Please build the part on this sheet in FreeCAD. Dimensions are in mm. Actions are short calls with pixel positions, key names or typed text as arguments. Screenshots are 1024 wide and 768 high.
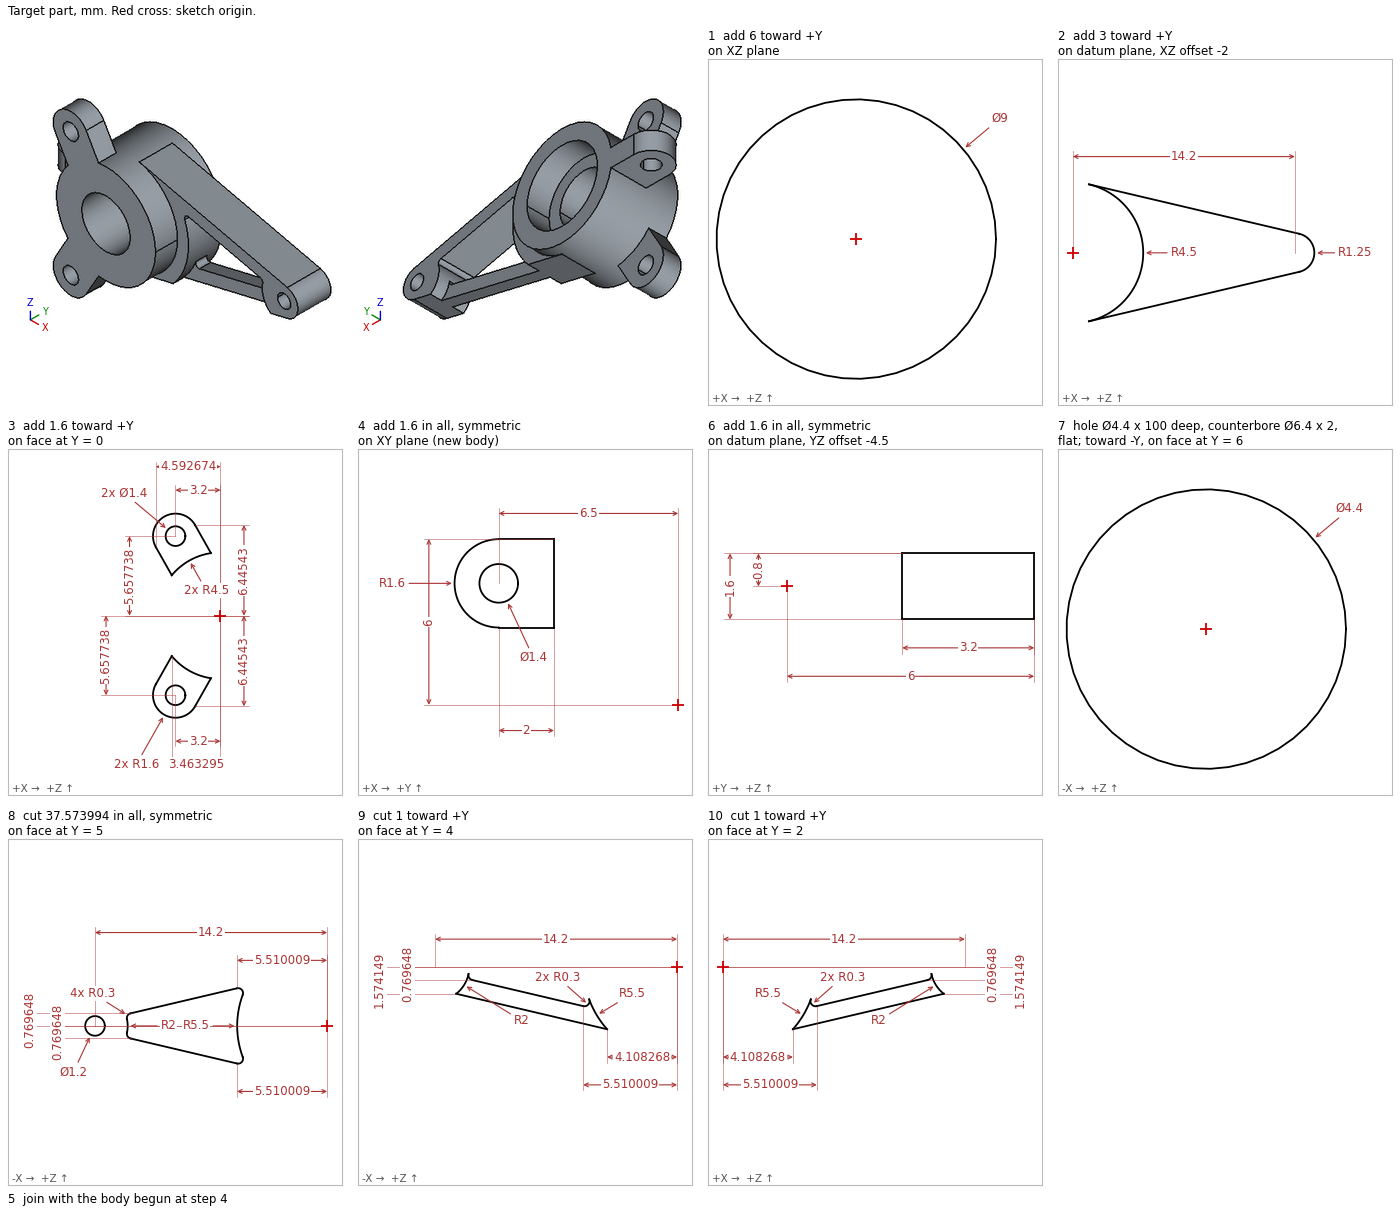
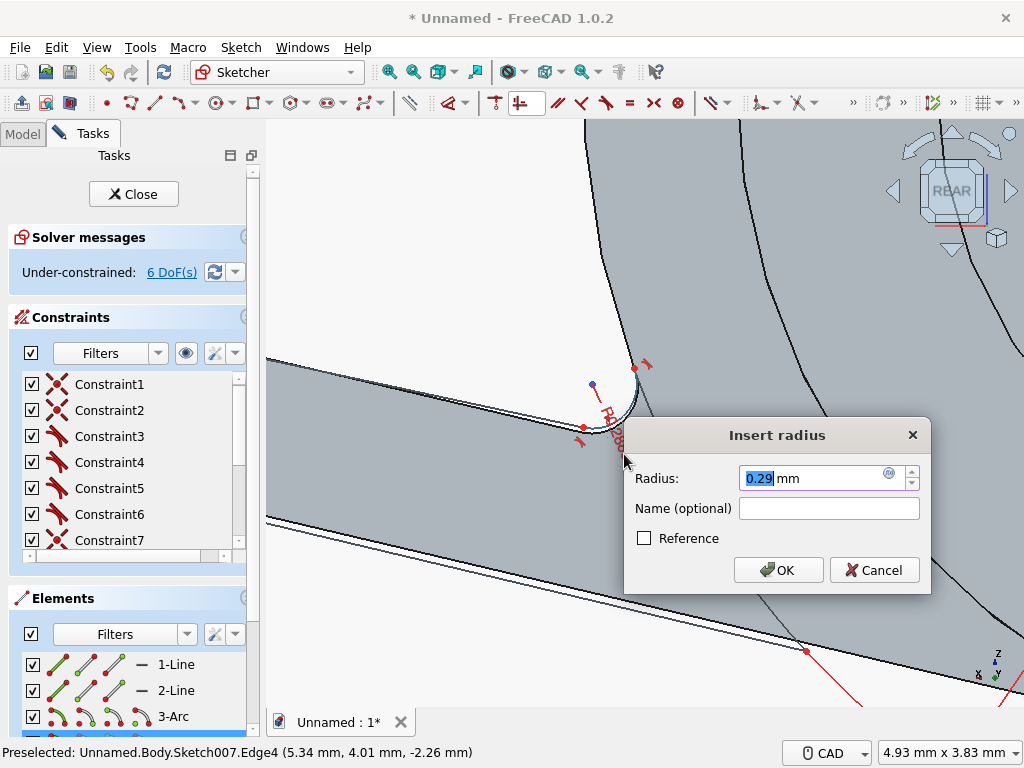
text(0.3)
key(Return)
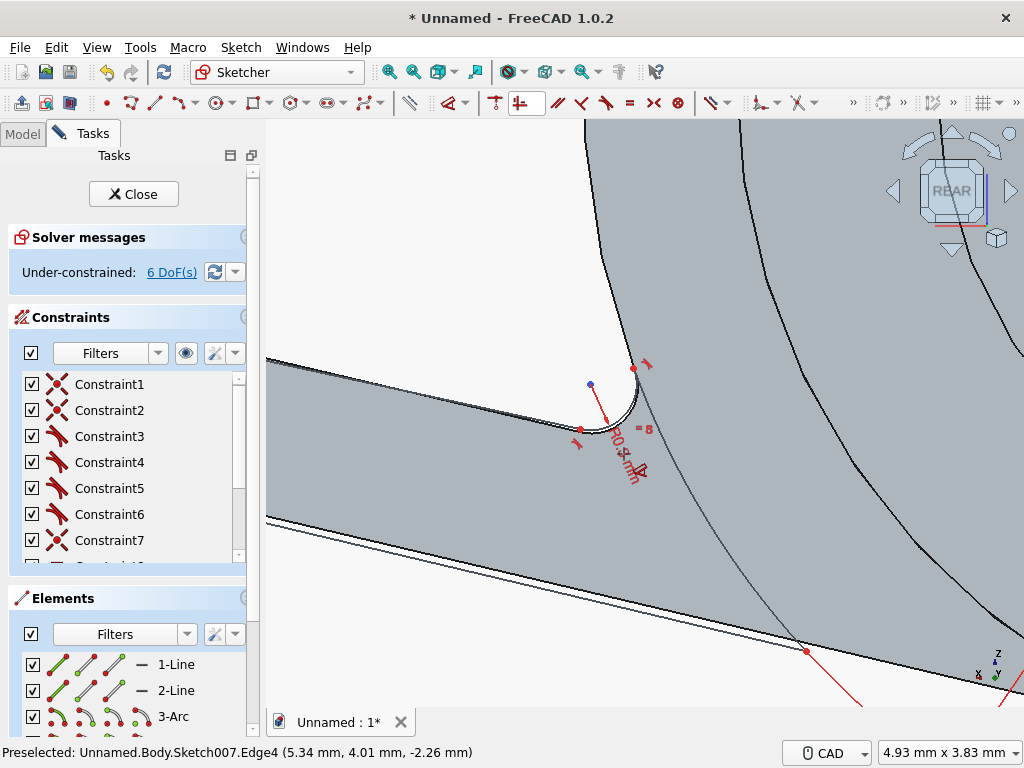
scroll(613, 426, down, 8)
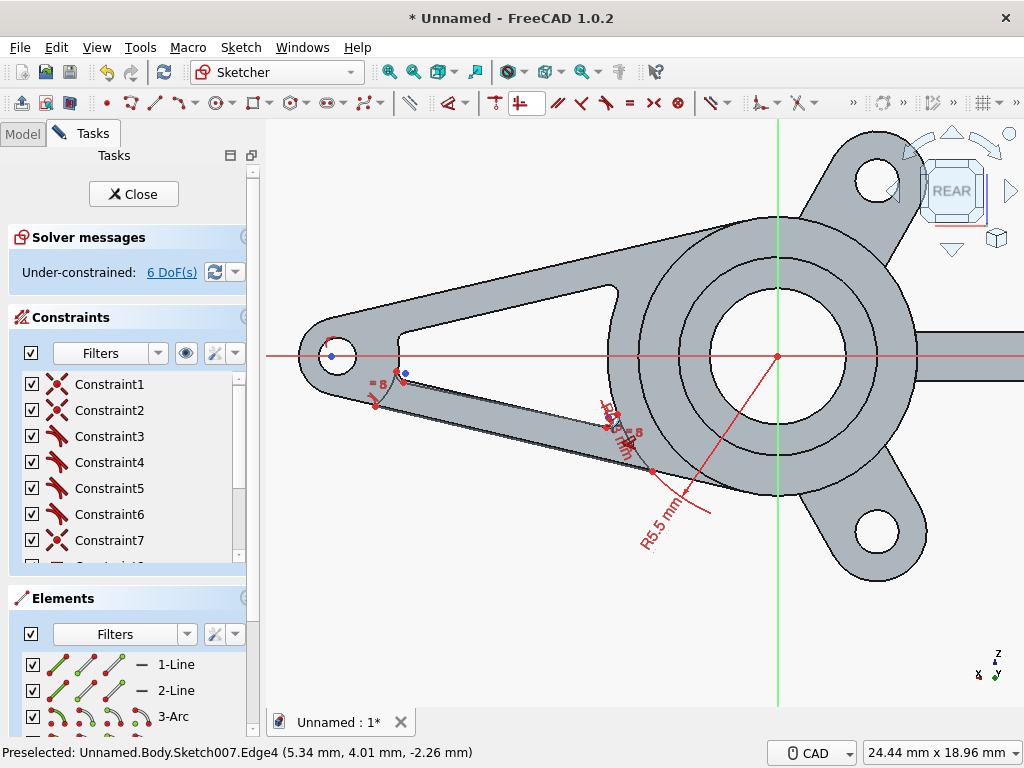
scroll(384, 397, up, 2)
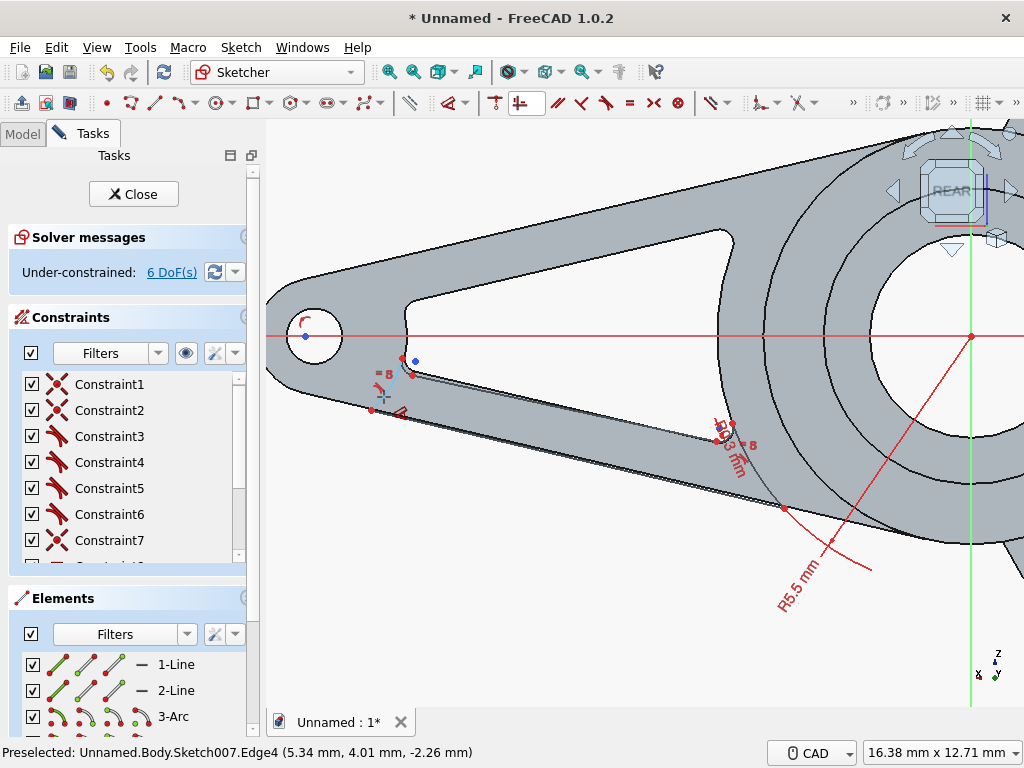
click(384, 397)
click(358, 457)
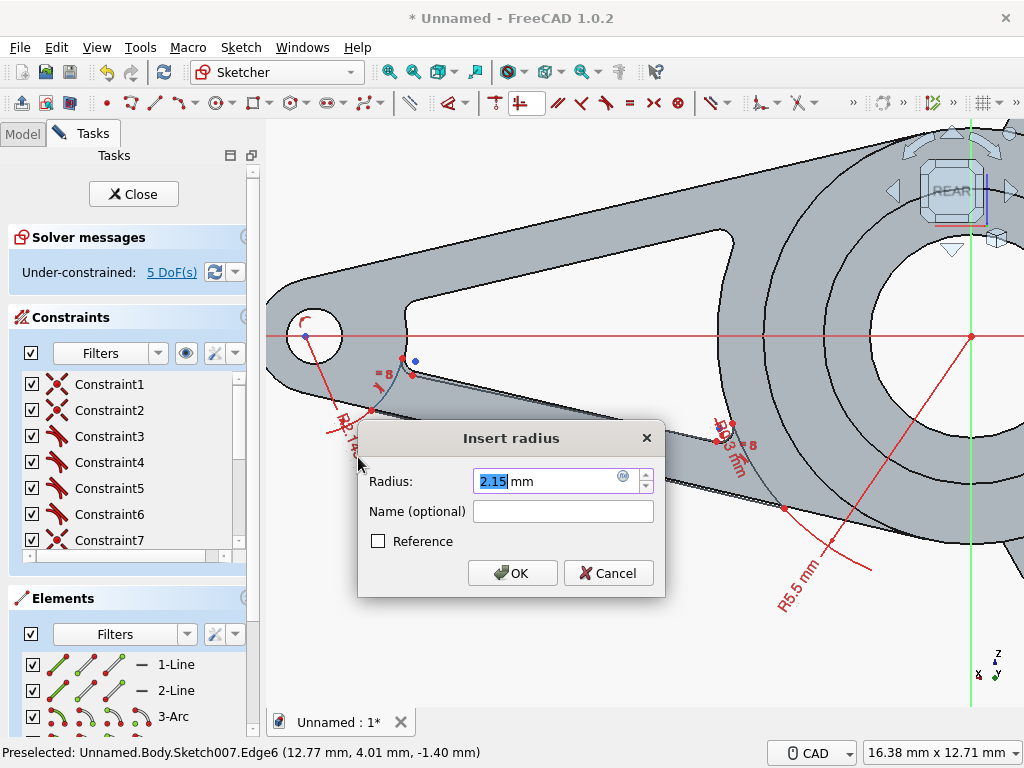
text(2)
key(Return)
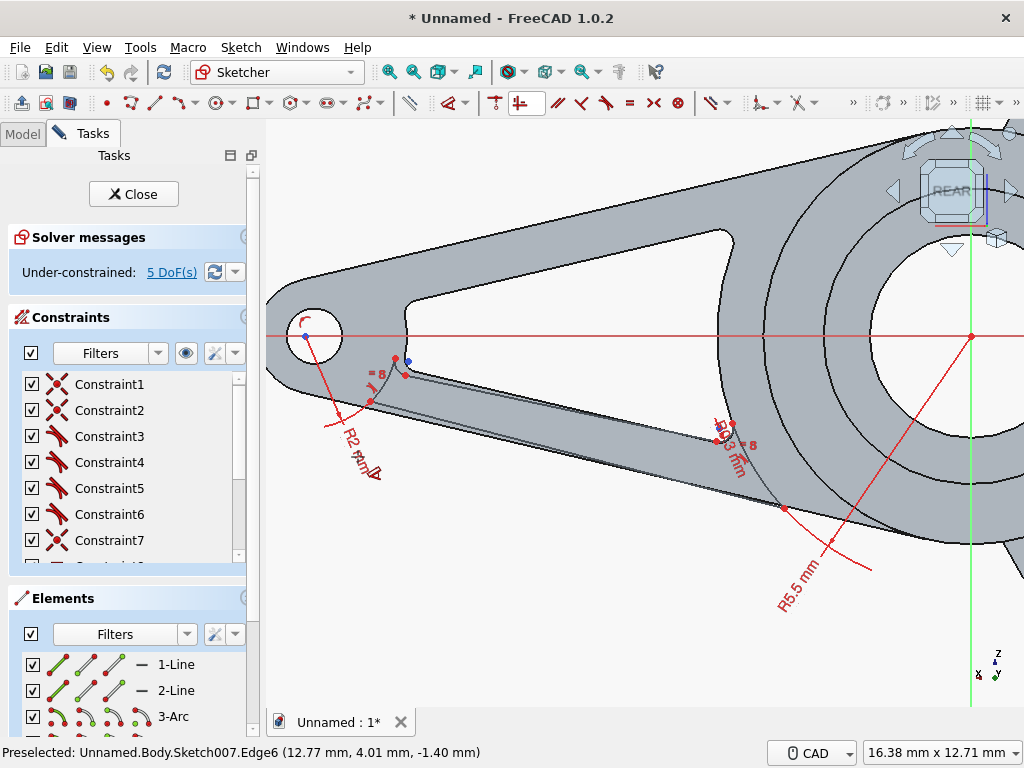
click(305, 336)
click(582, 302)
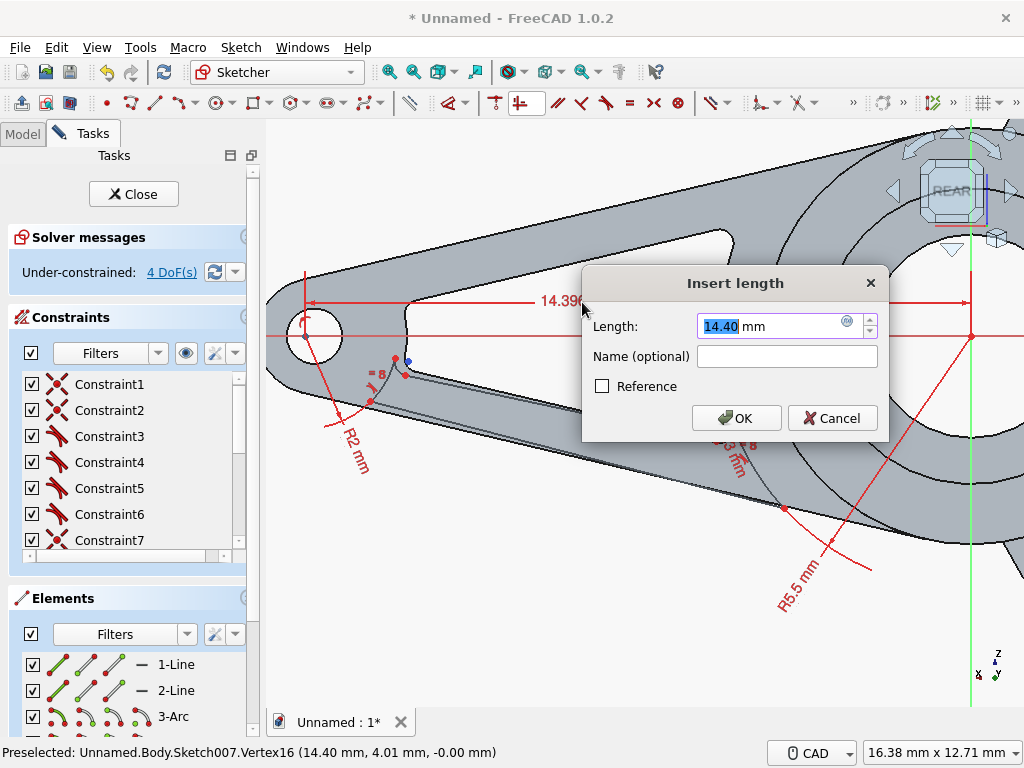
text(14.2)
key(Return)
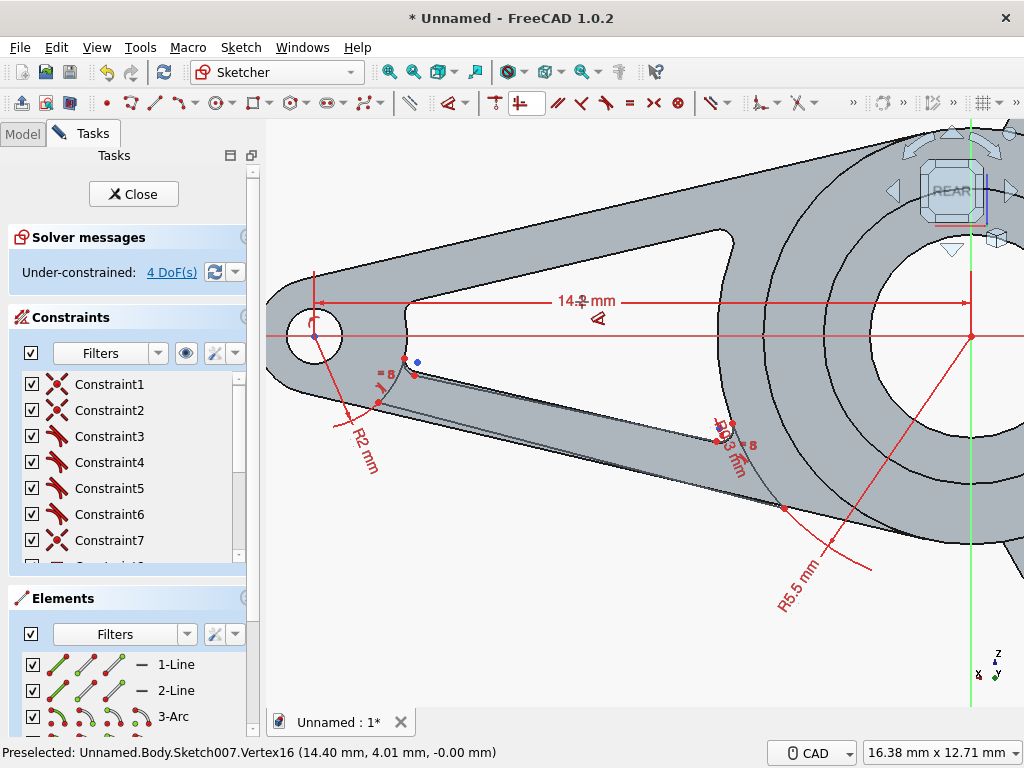
click(379, 403)
click(345, 369)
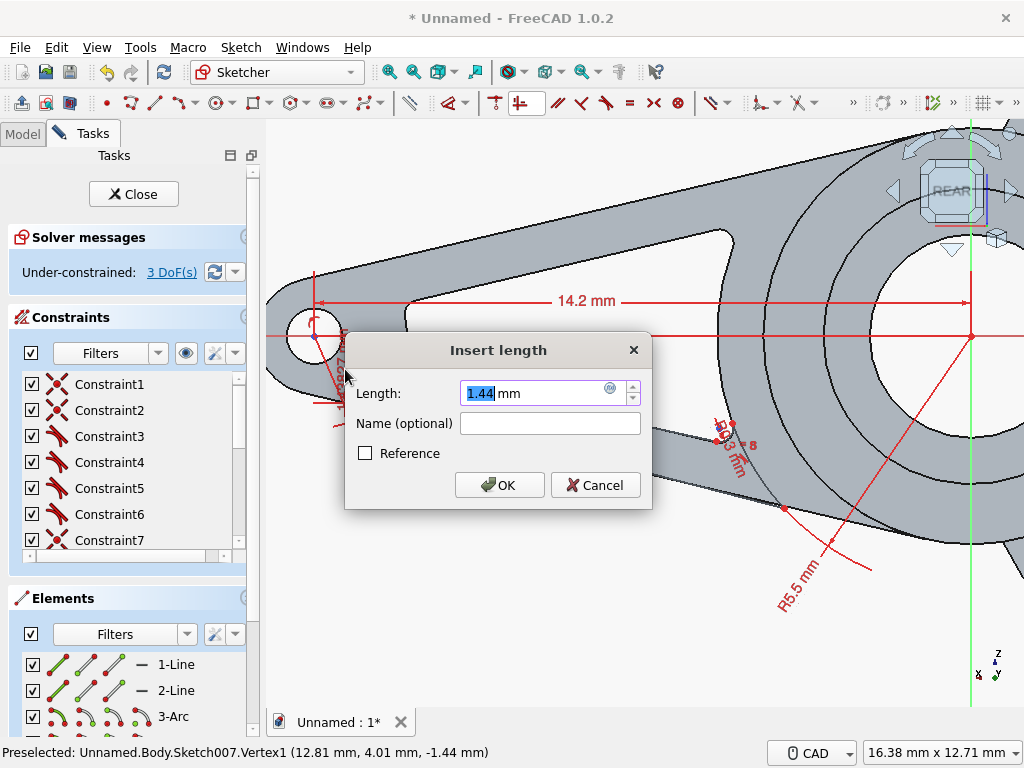
text(1.574149)
key(Return)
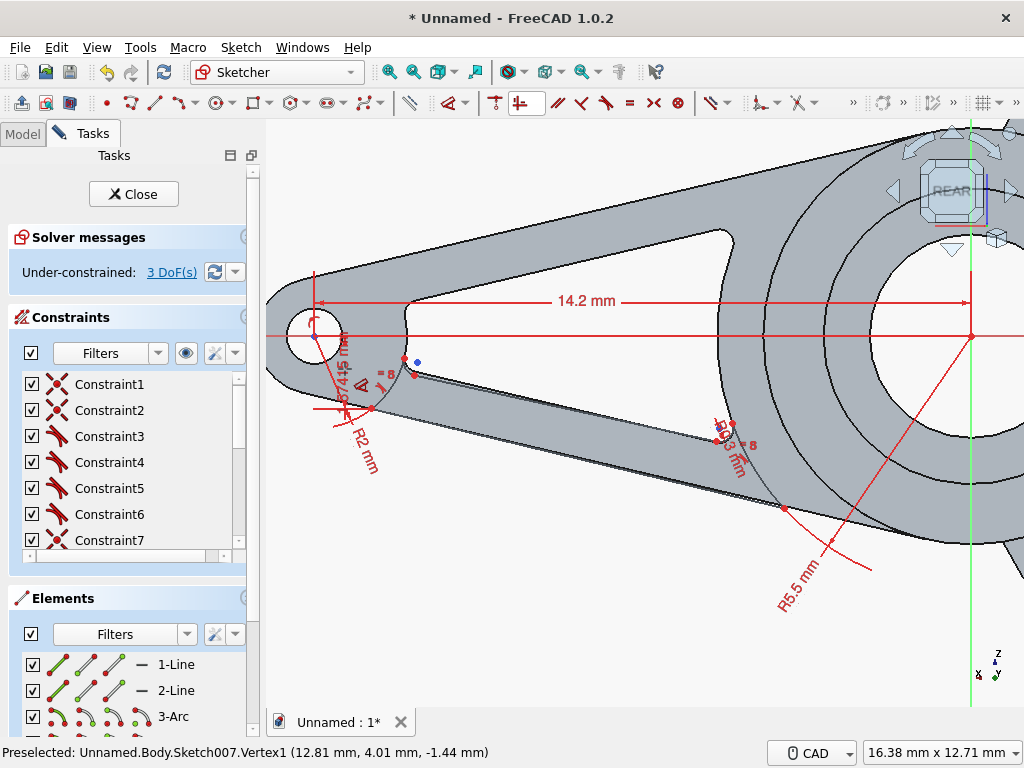
click(784, 509)
click(822, 543)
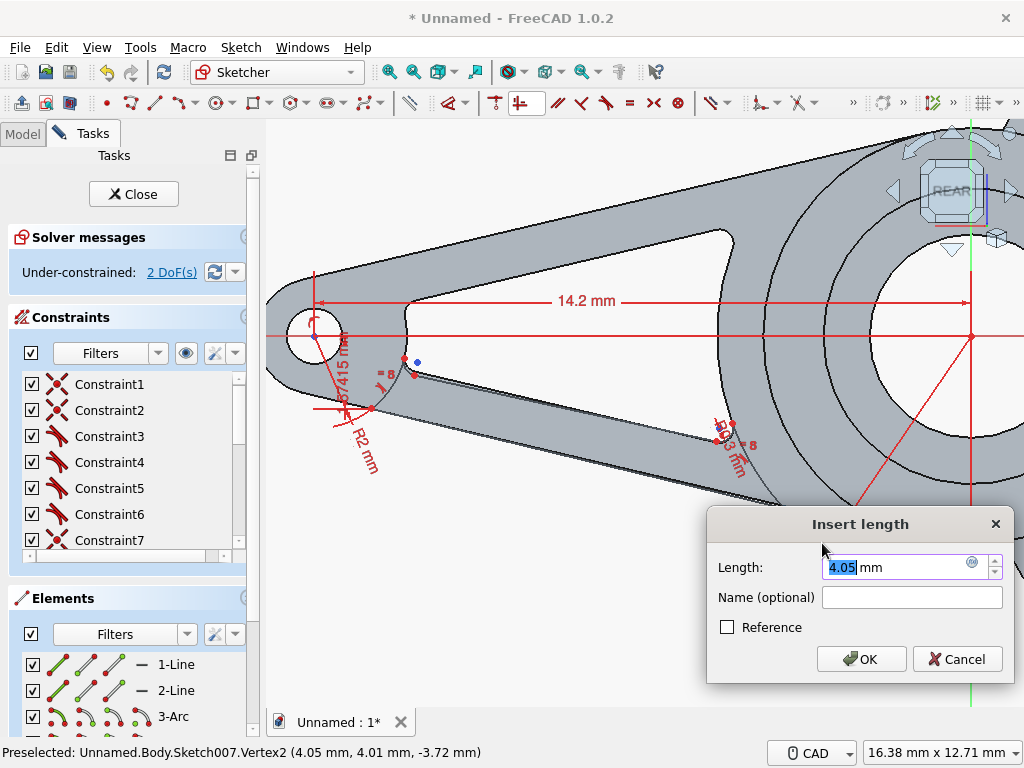
text(4.108268)
key(Return)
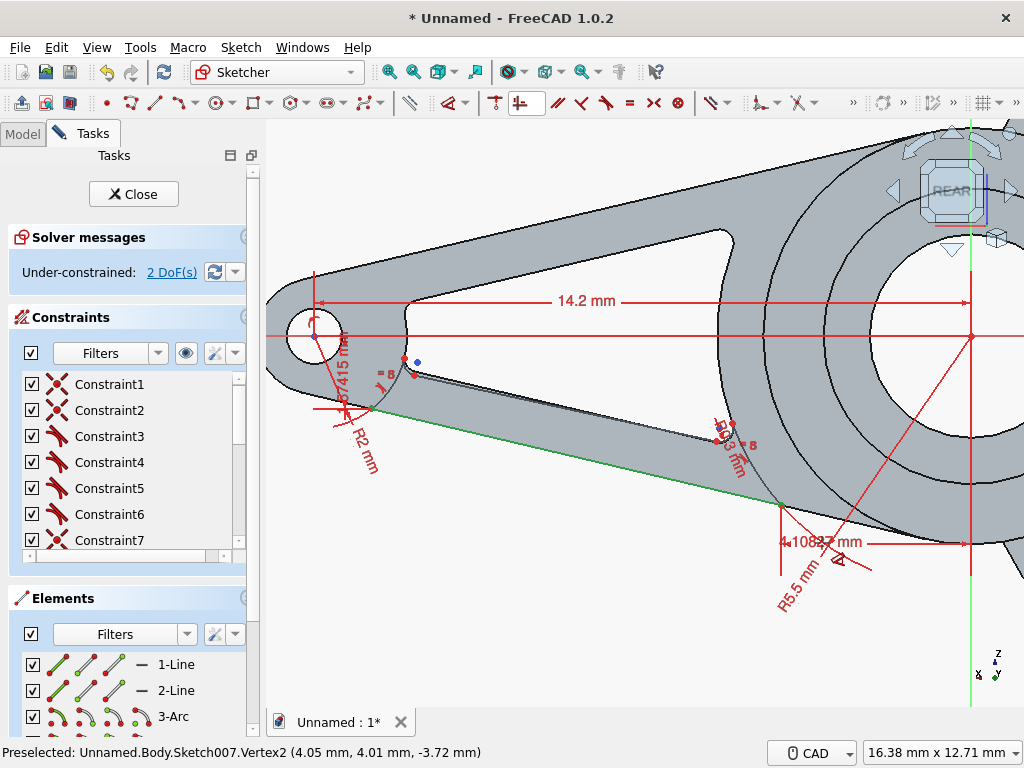
click(716, 442)
click(788, 302)